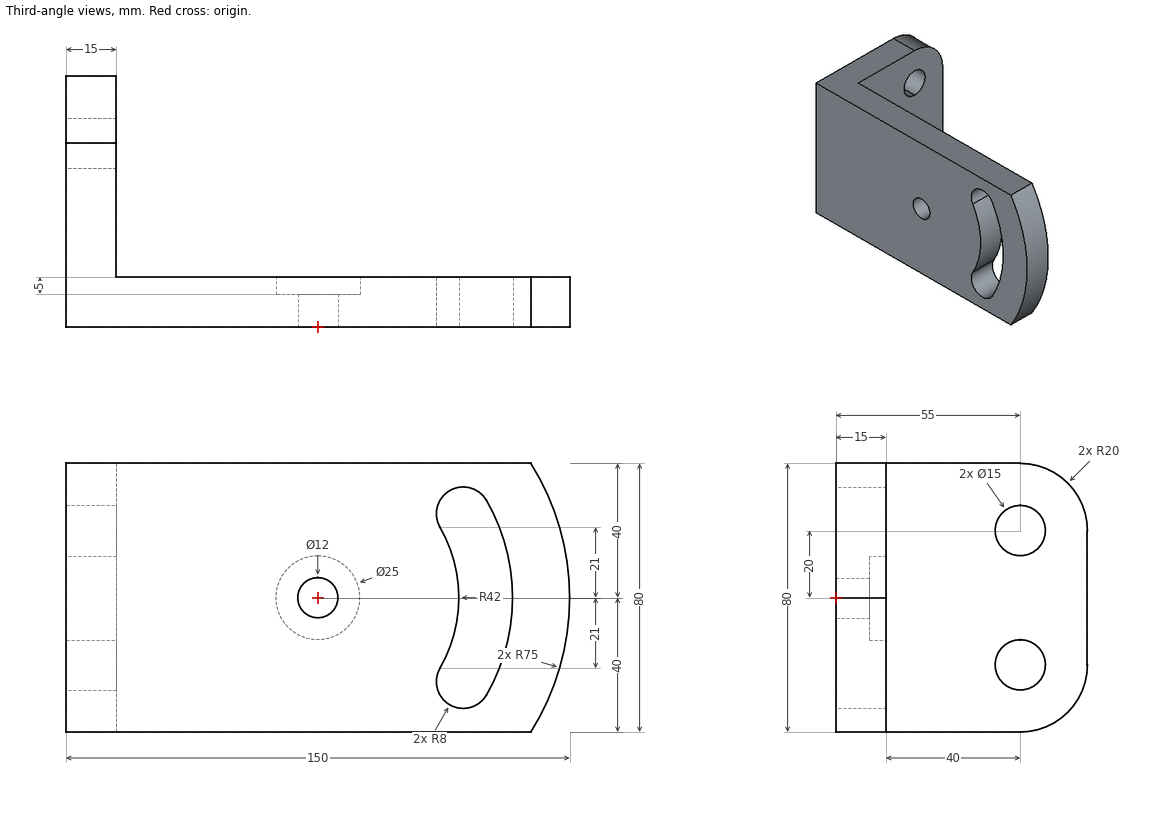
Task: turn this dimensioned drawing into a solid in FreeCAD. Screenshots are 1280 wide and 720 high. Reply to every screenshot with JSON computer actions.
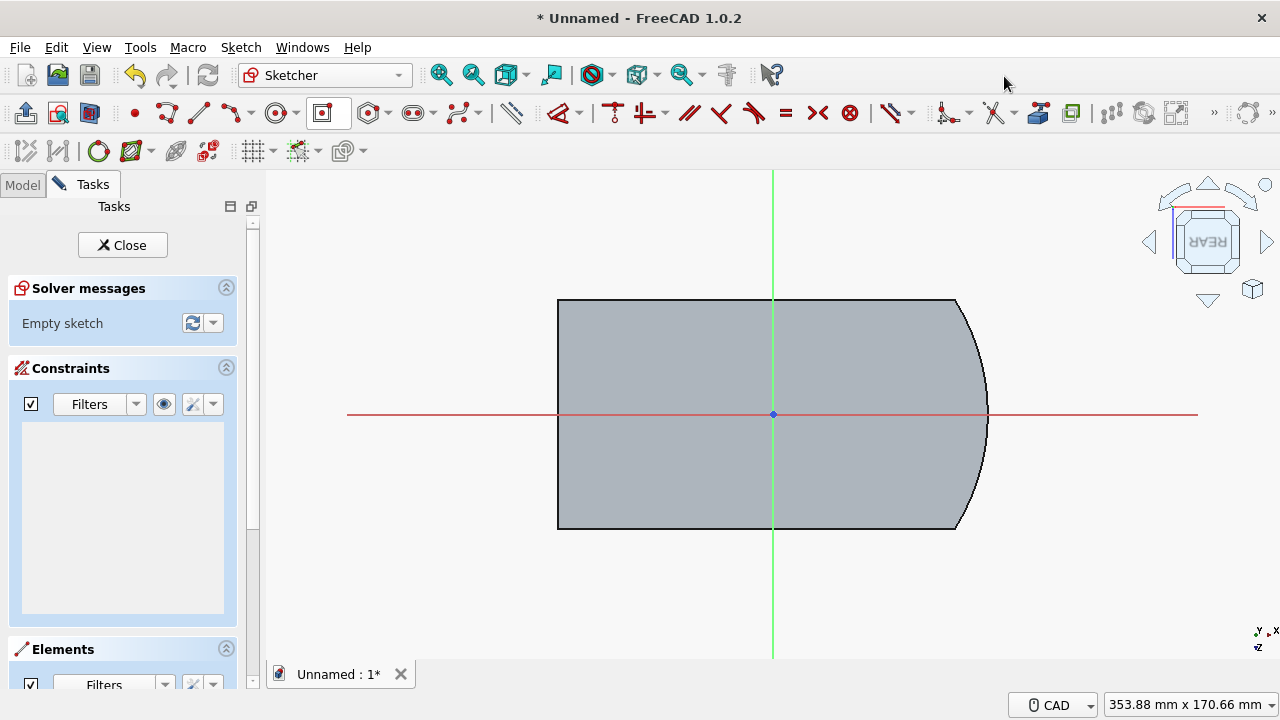
{"action": "scroll", "coordinate": [795, 414], "scroll_direction": "up", "scroll_amount": 7}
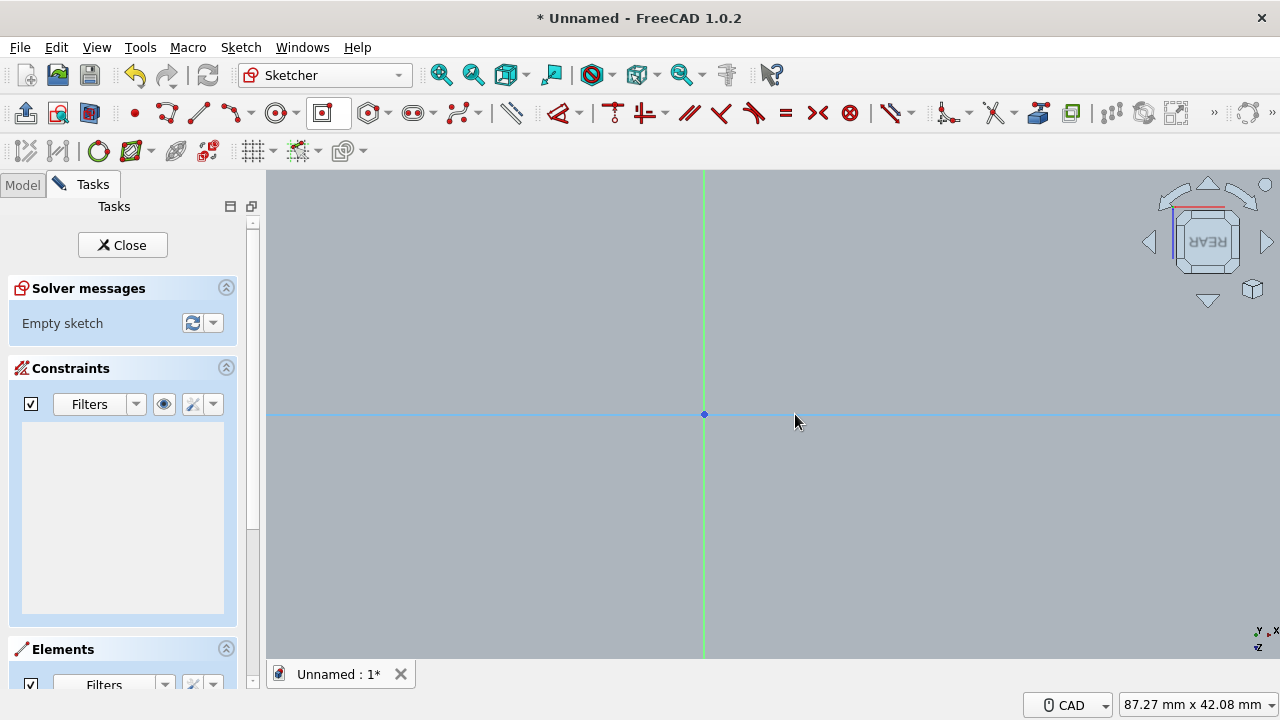
{"action": "left_click", "coordinate": [276, 114]}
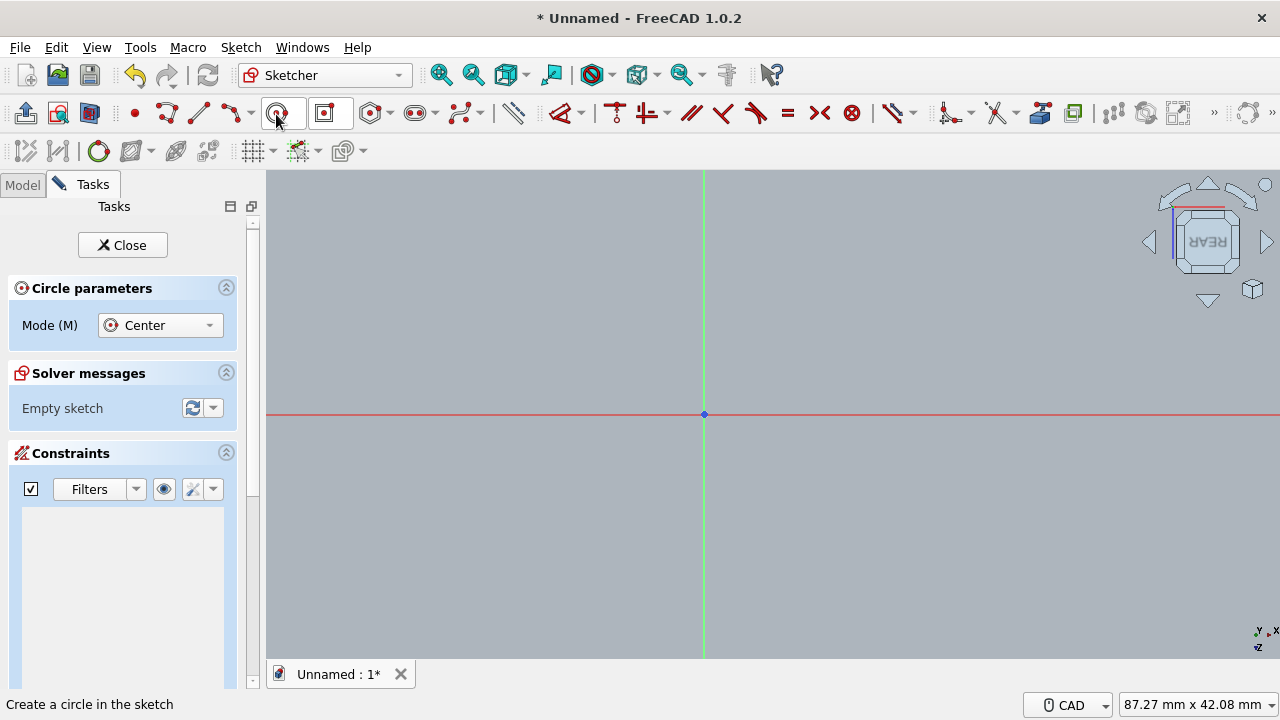
{"action": "left_click", "coordinate": [704, 414]}
{"action": "left_click", "coordinate": [807, 312]}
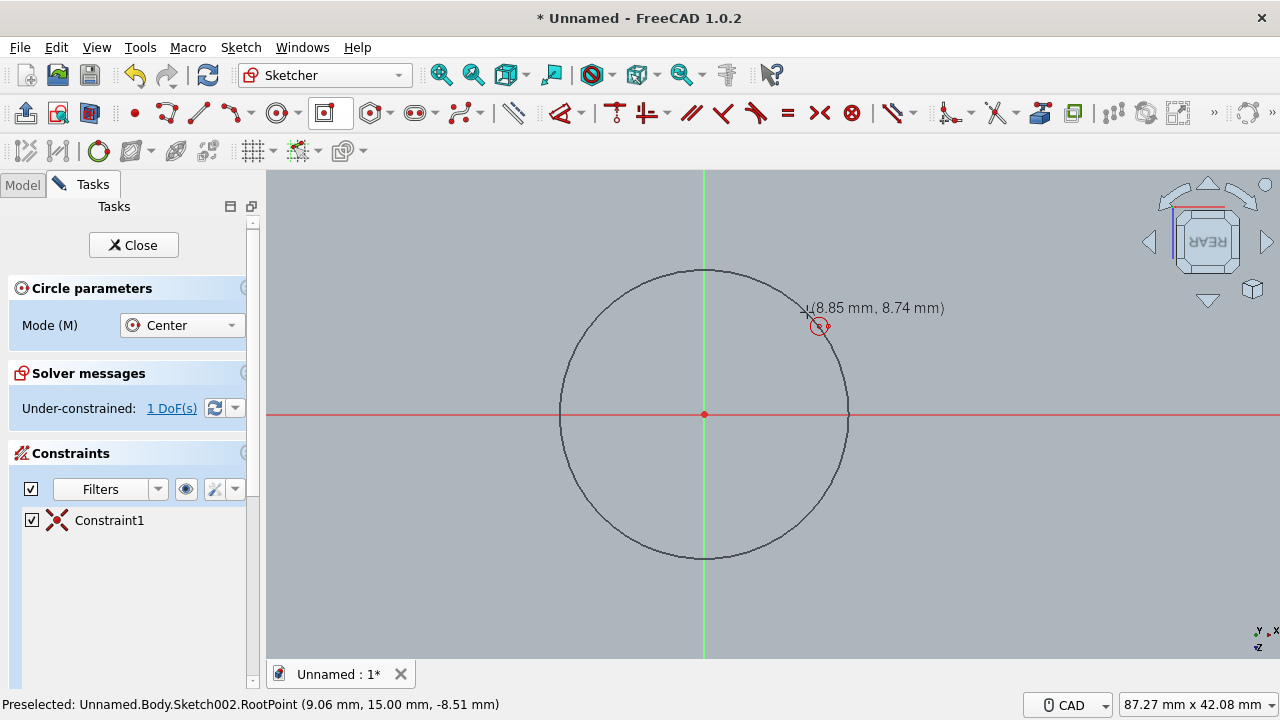
{"action": "left_click", "coordinate": [704, 414]}
{"action": "left_click", "coordinate": [753, 365]}
{"action": "key", "text": "Escape"}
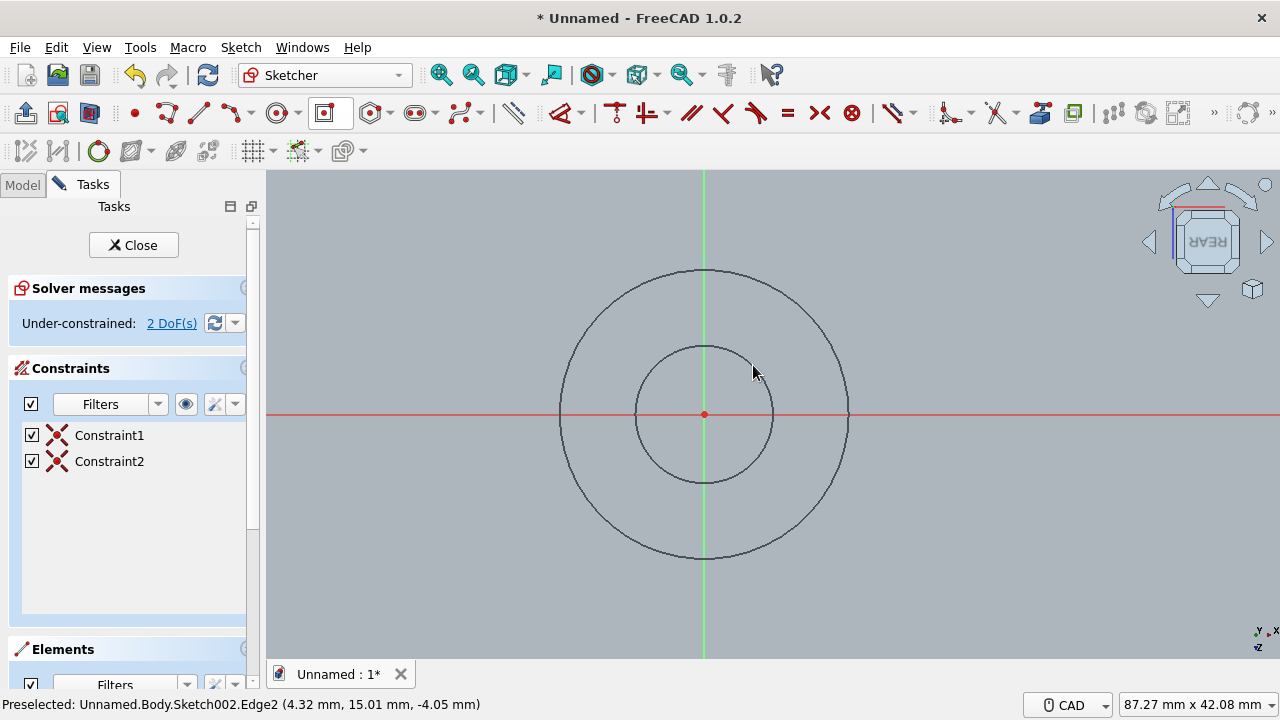
{"action": "left_click", "coordinate": [560, 114]}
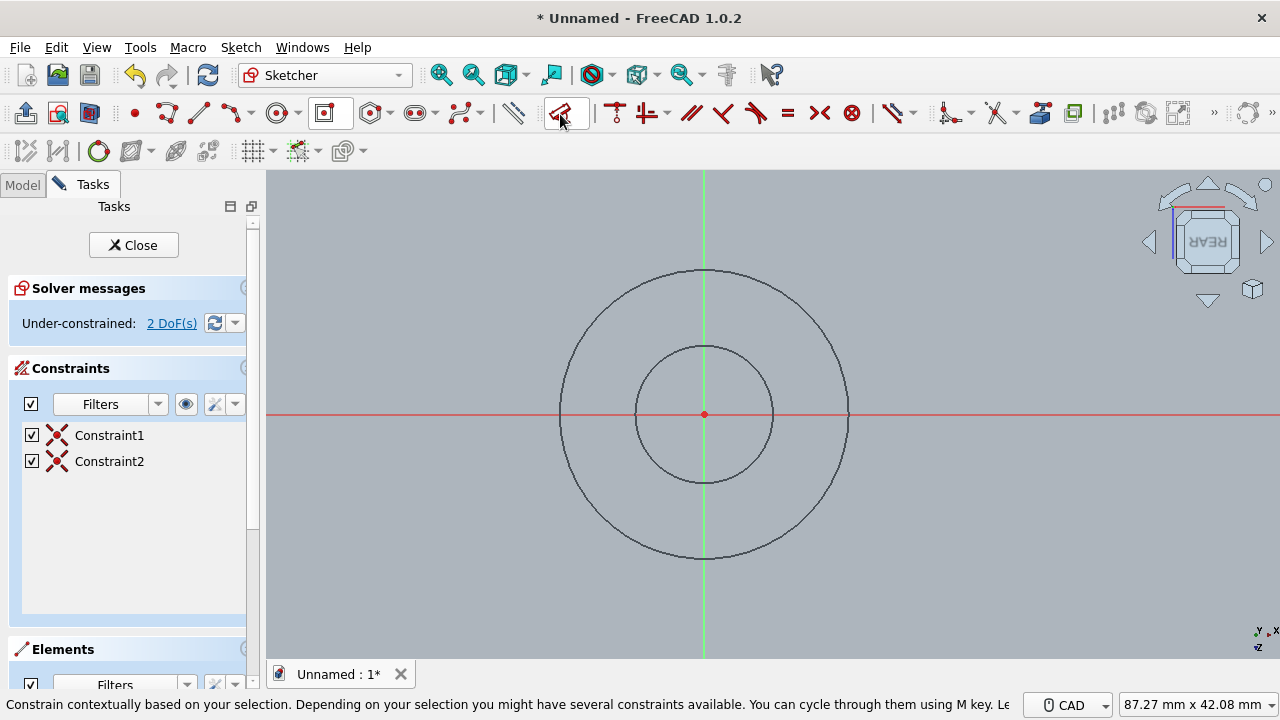
{"action": "left_click", "coordinate": [806, 312]}
{"action": "left_click", "coordinate": [829, 289]}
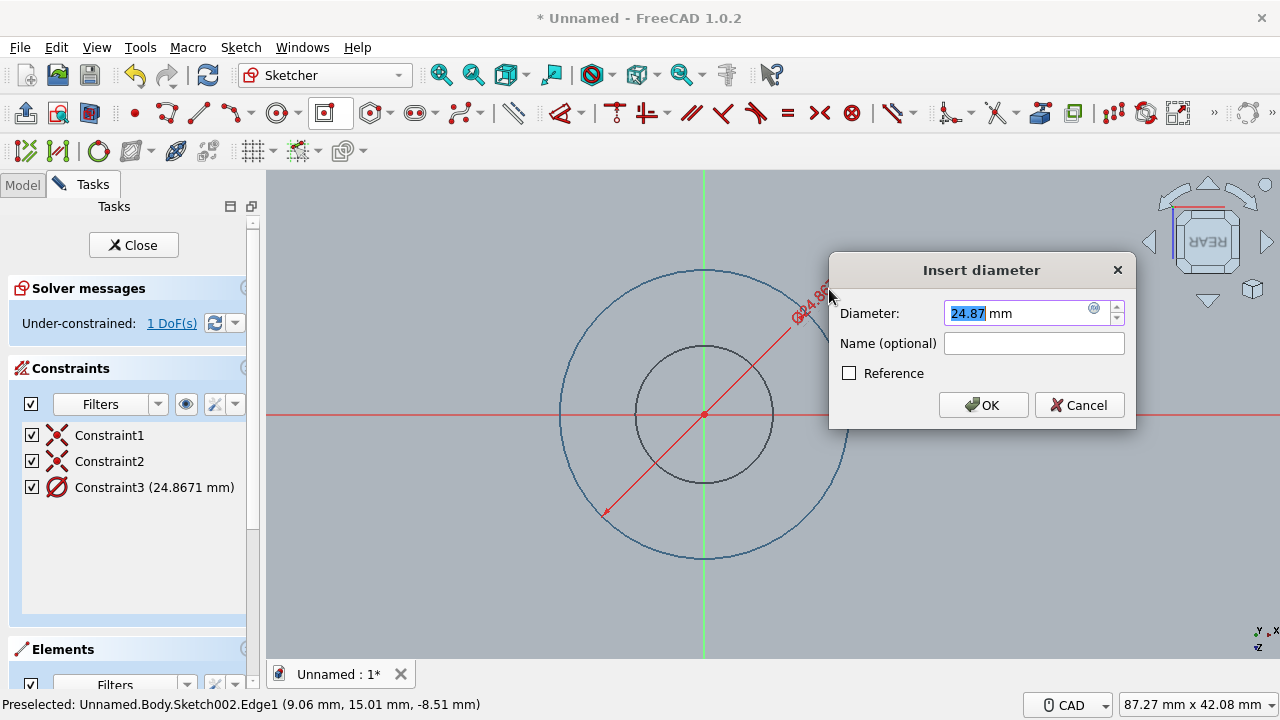
{"action": "type", "text": "25"}
{"action": "key", "text": "Return"}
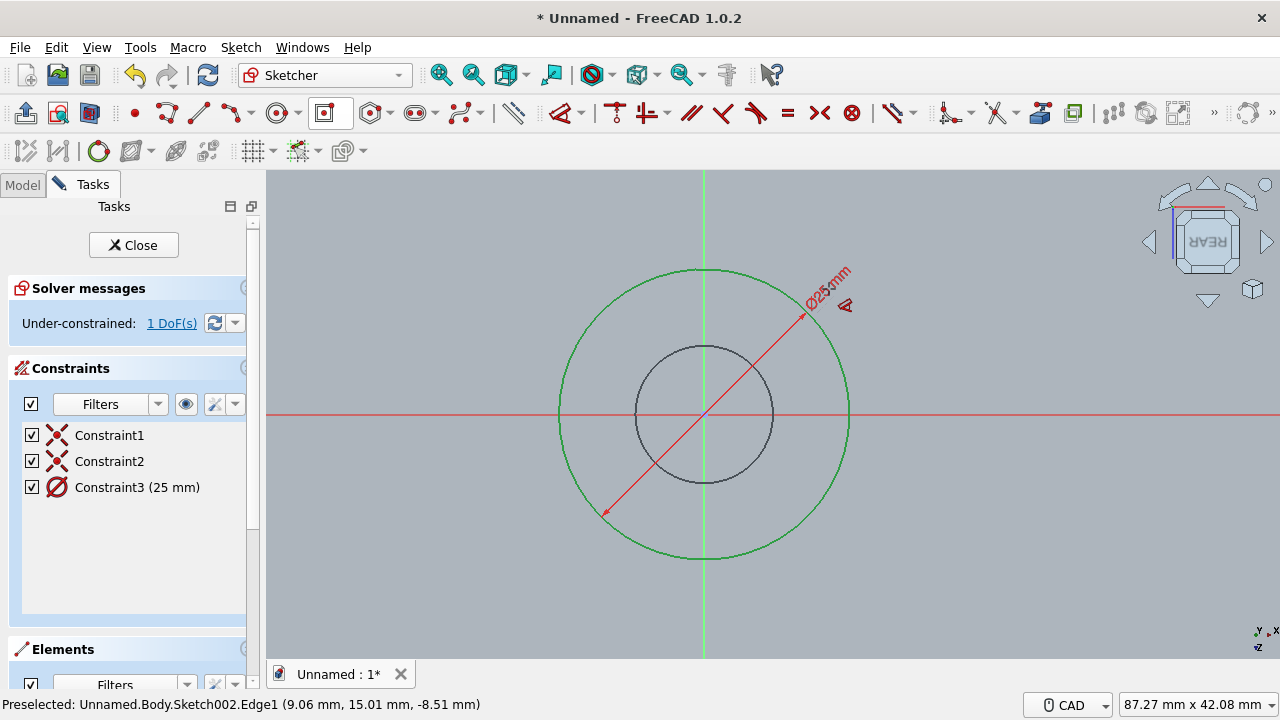
{"action": "left_click", "coordinate": [753, 366]}
{"action": "left_click", "coordinate": [776, 343]}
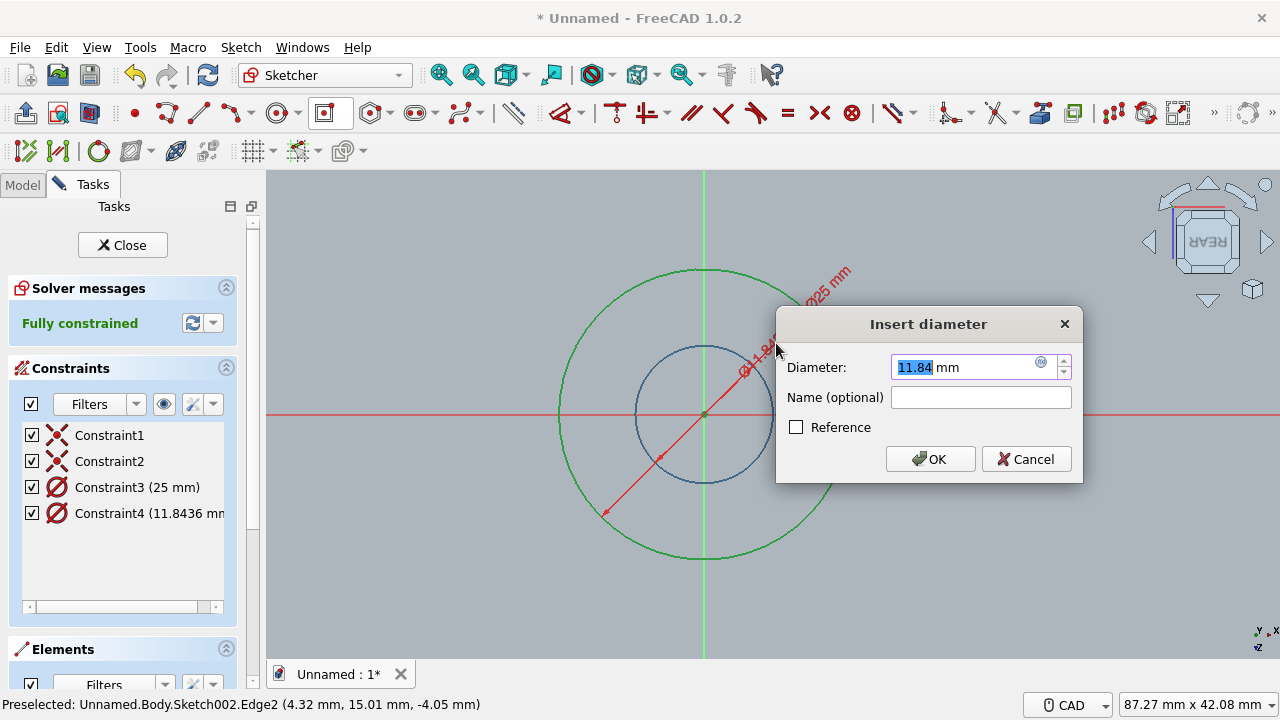
{"action": "type", "text": "12"}
{"action": "key", "text": "Return"}
{"action": "key", "text": "Escape"}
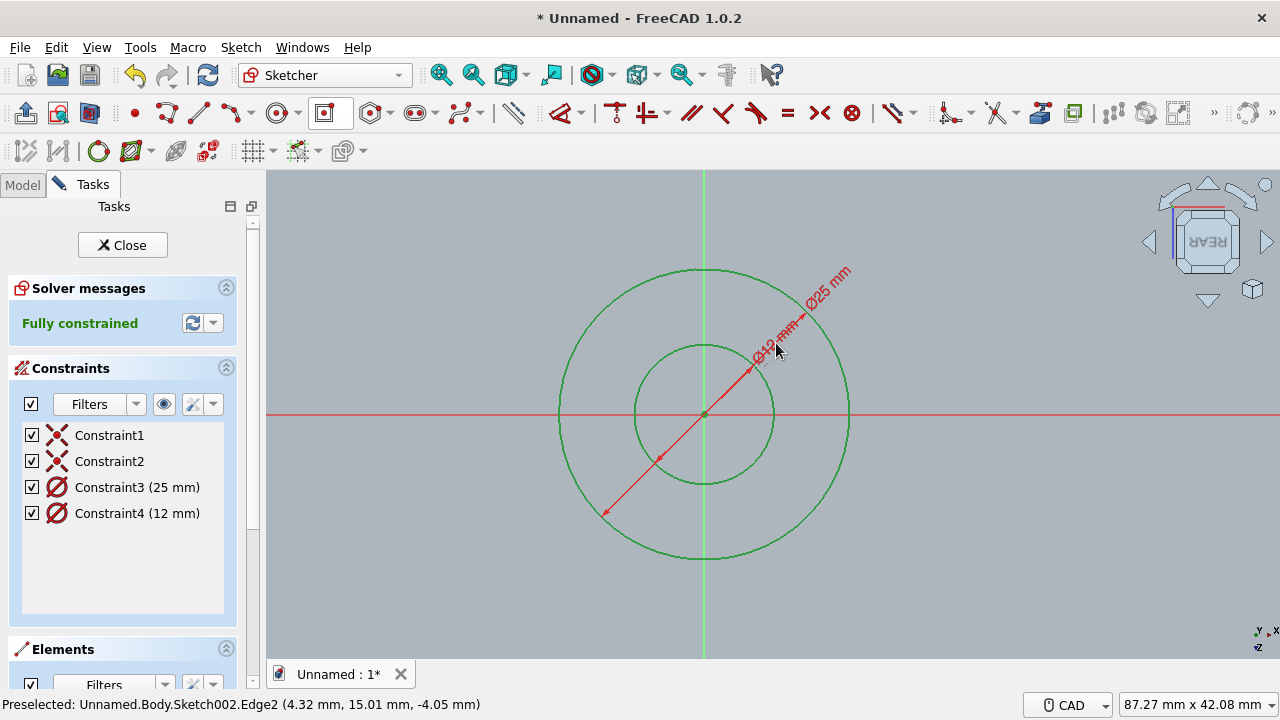
{"action": "left_click", "coordinate": [123, 245]}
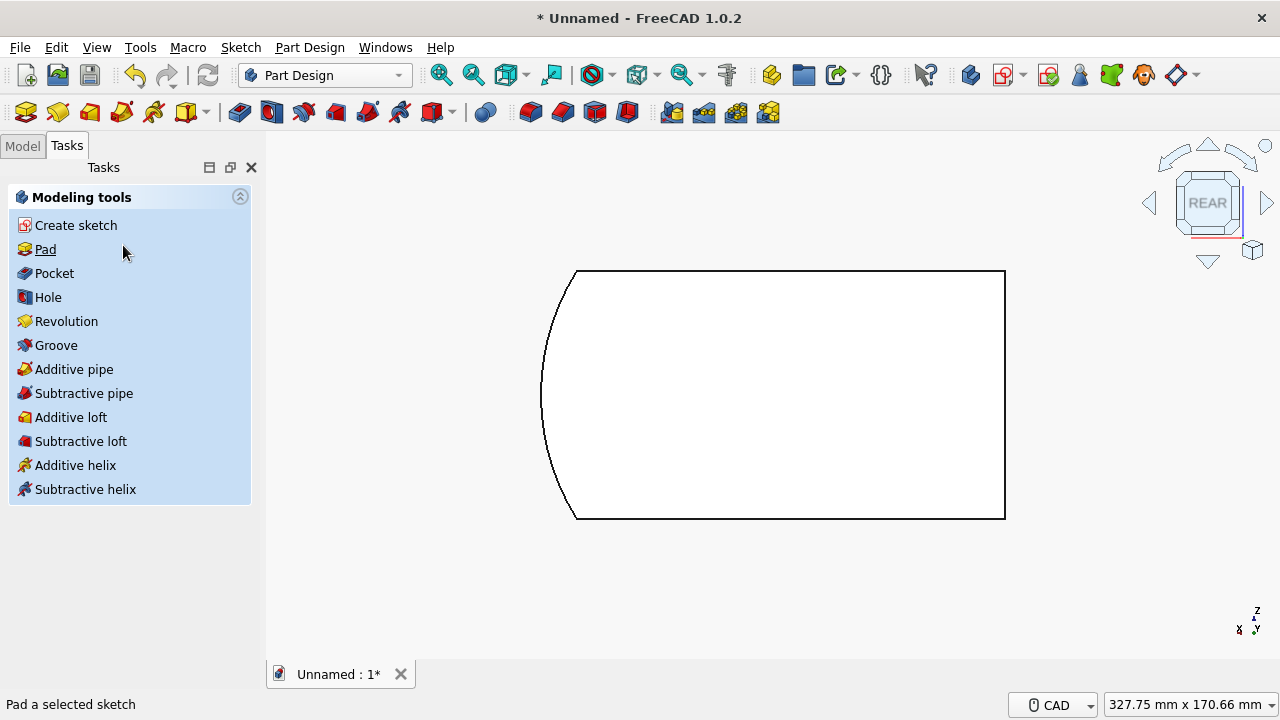
{"action": "left_click", "coordinate": [240, 112]}